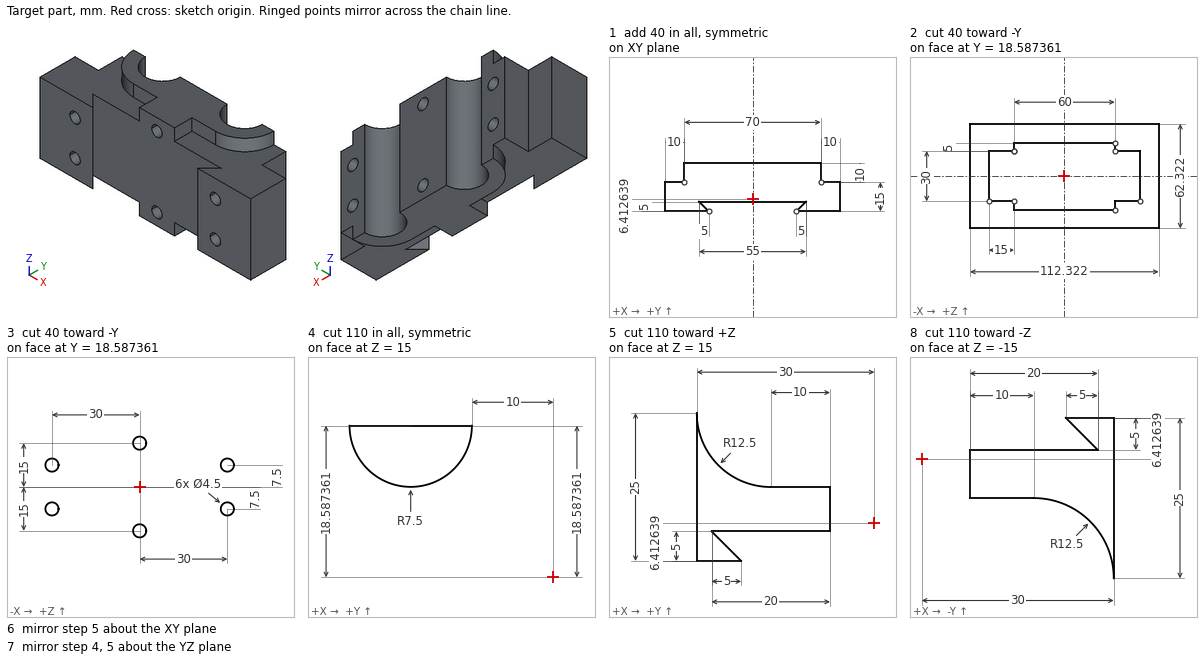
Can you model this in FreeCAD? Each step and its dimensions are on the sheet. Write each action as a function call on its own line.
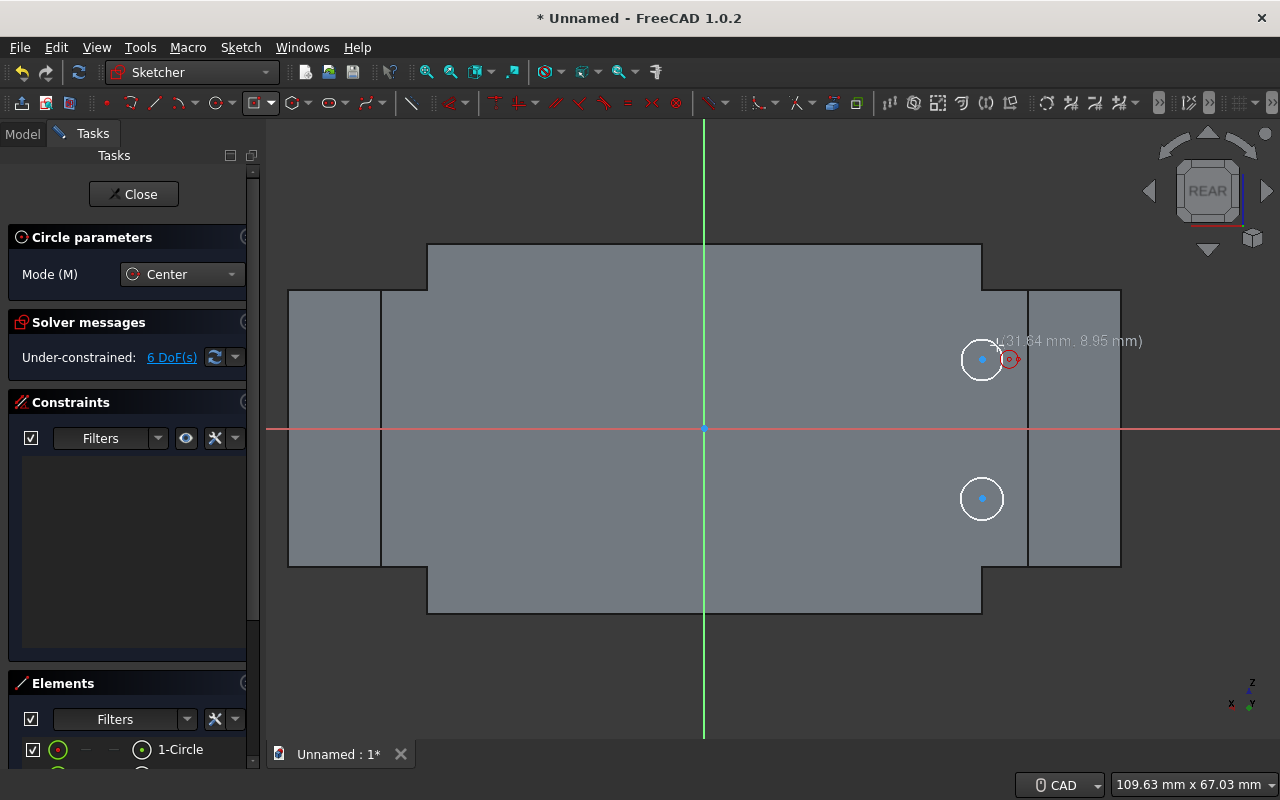
click(427, 359)
click(442, 345)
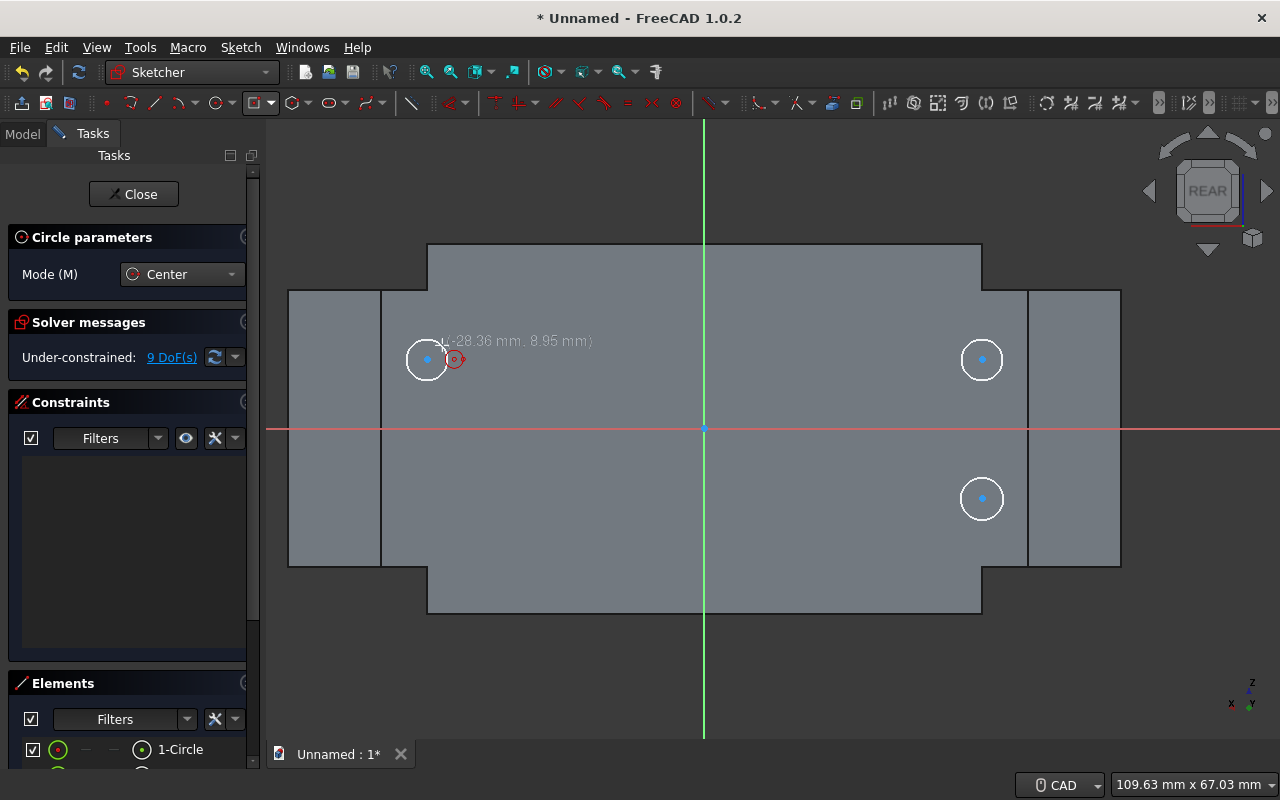
click(427, 498)
click(442, 483)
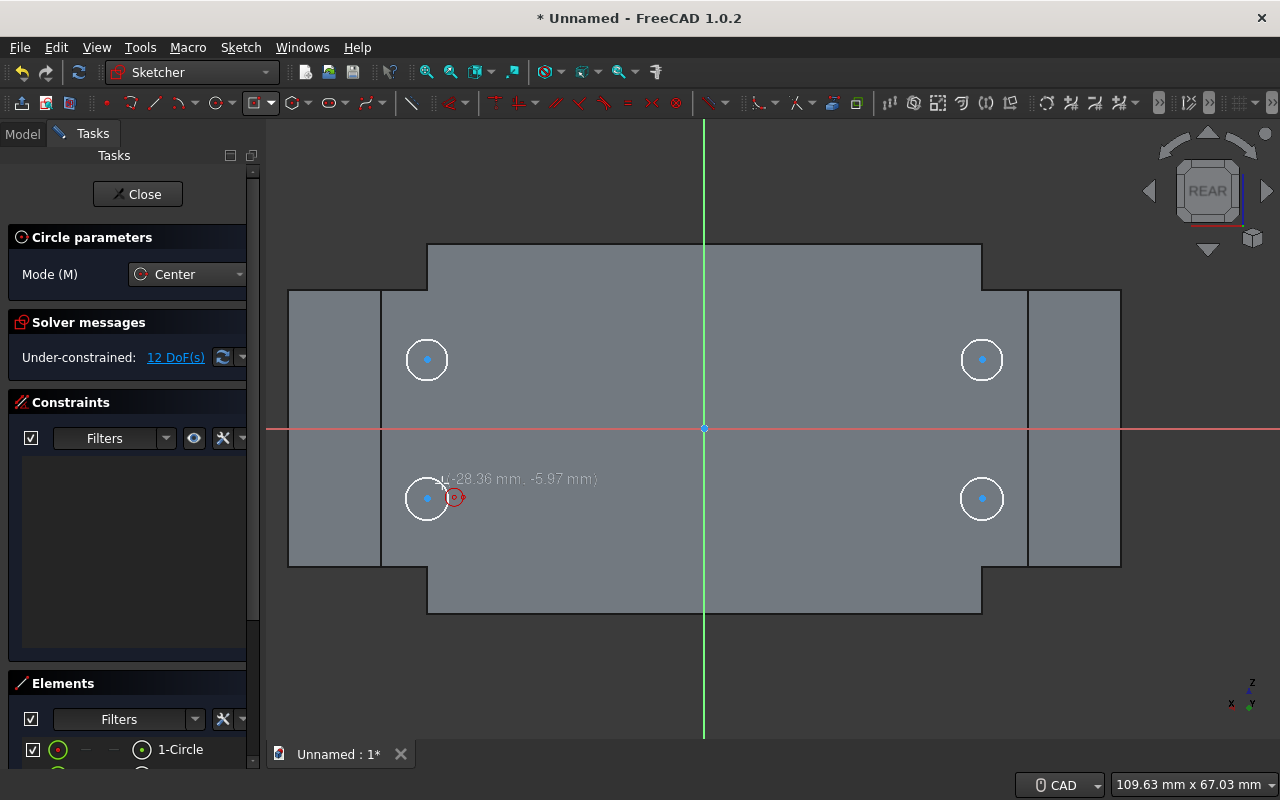
click(704, 567)
click(719, 553)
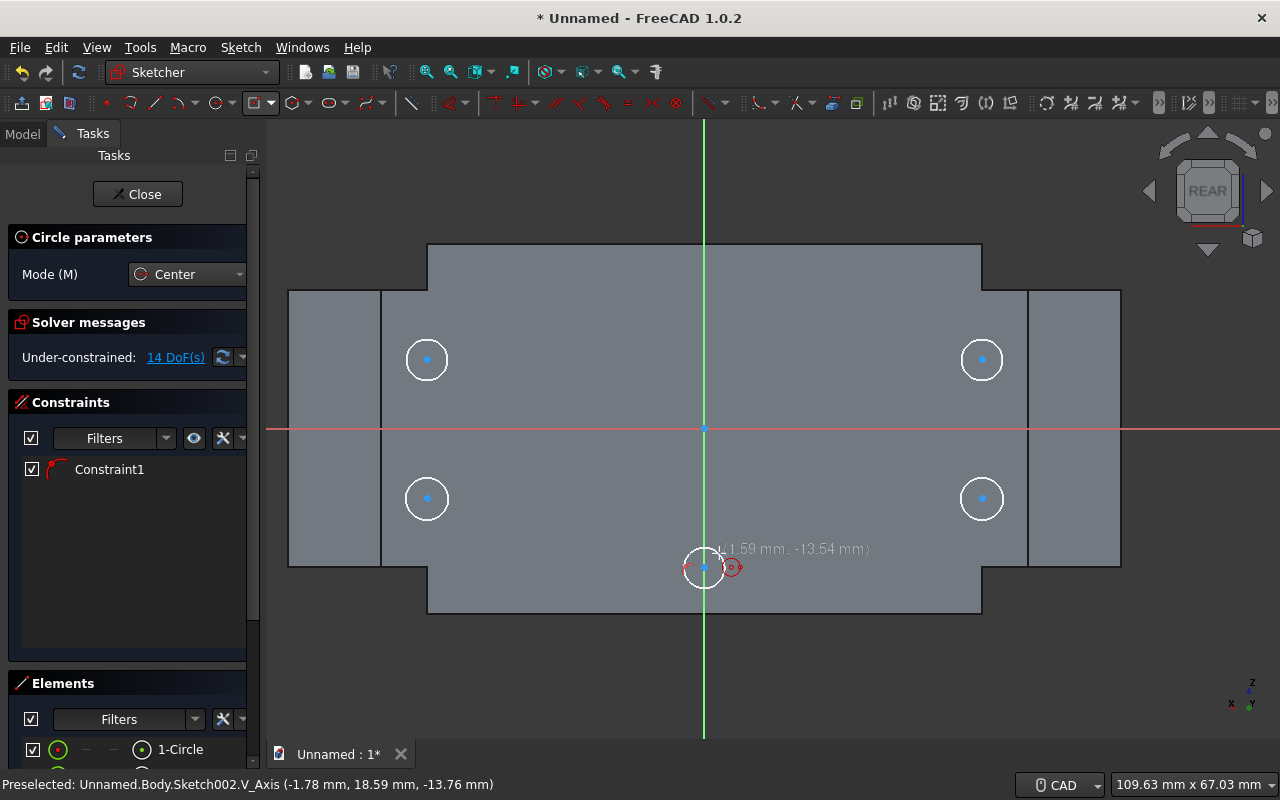
click(704, 290)
click(719, 275)
key(Escape)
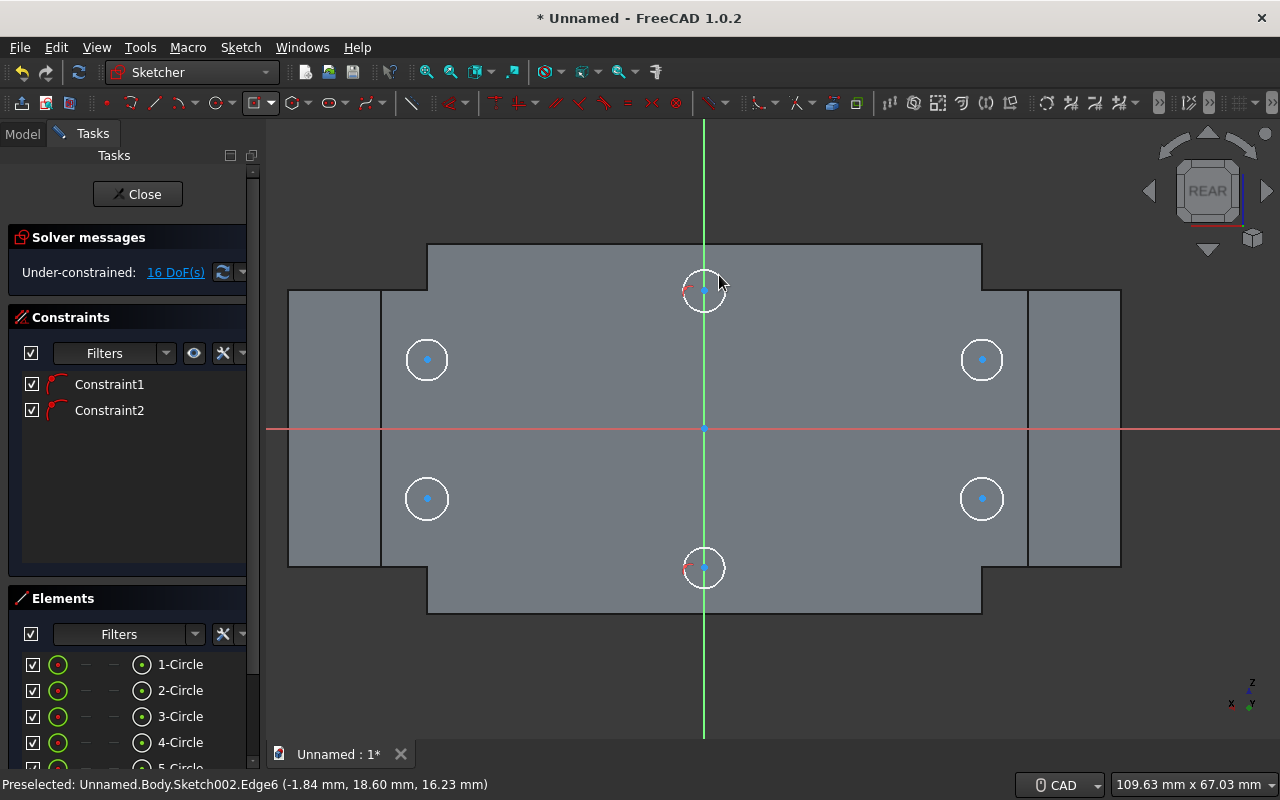
click(997, 484)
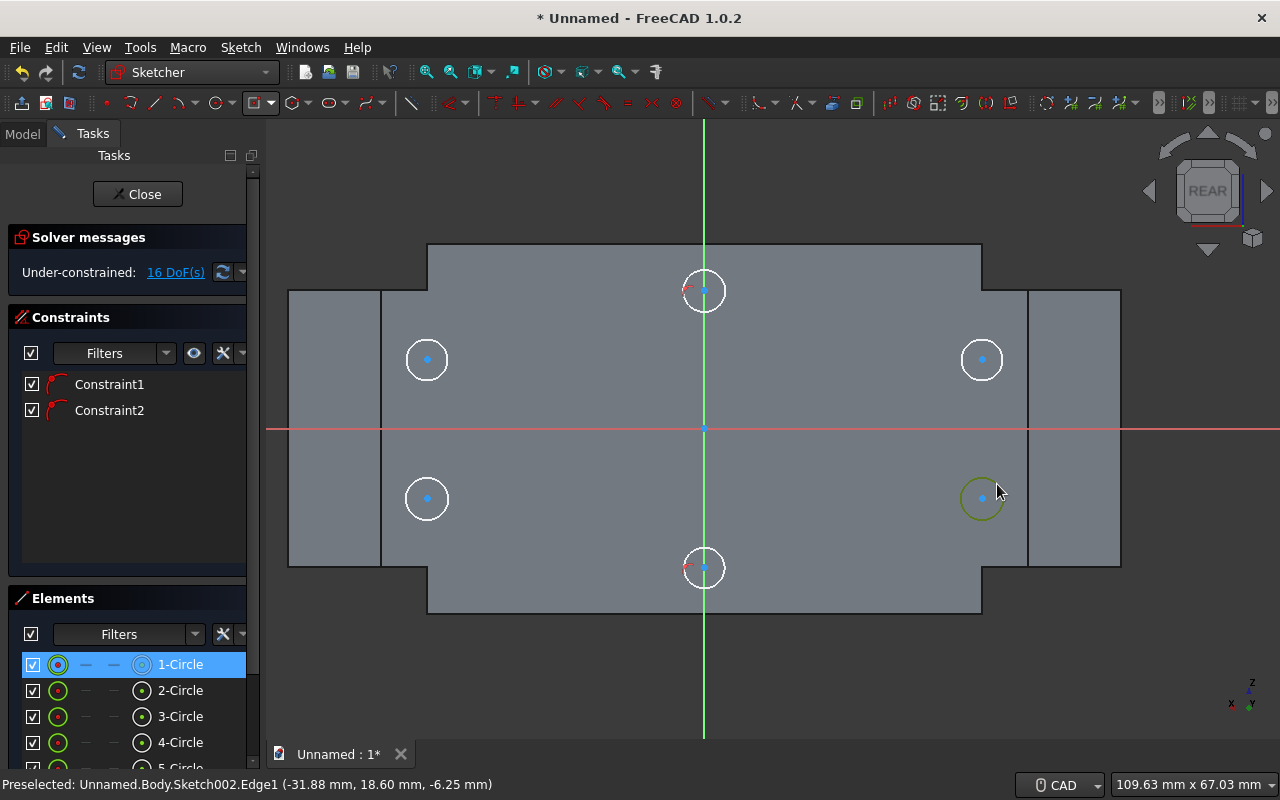
click(996, 345)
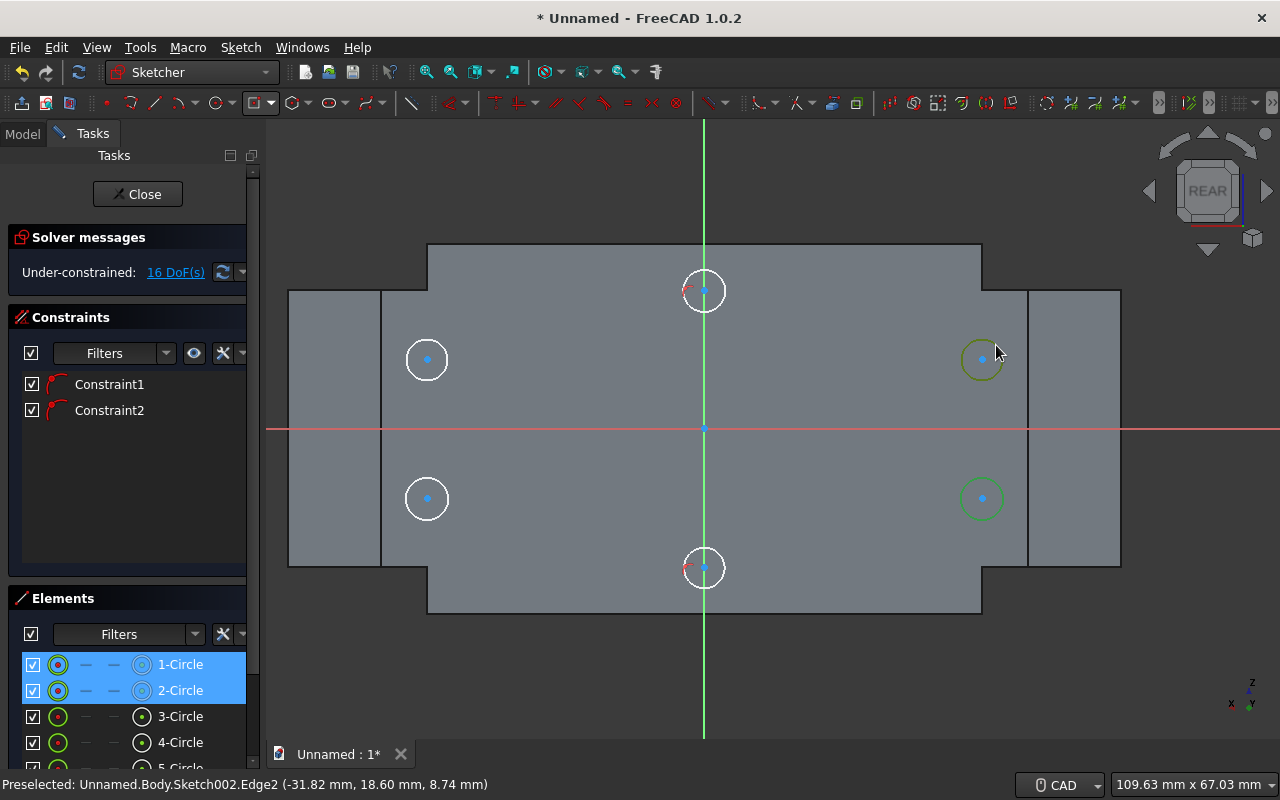
click(441, 345)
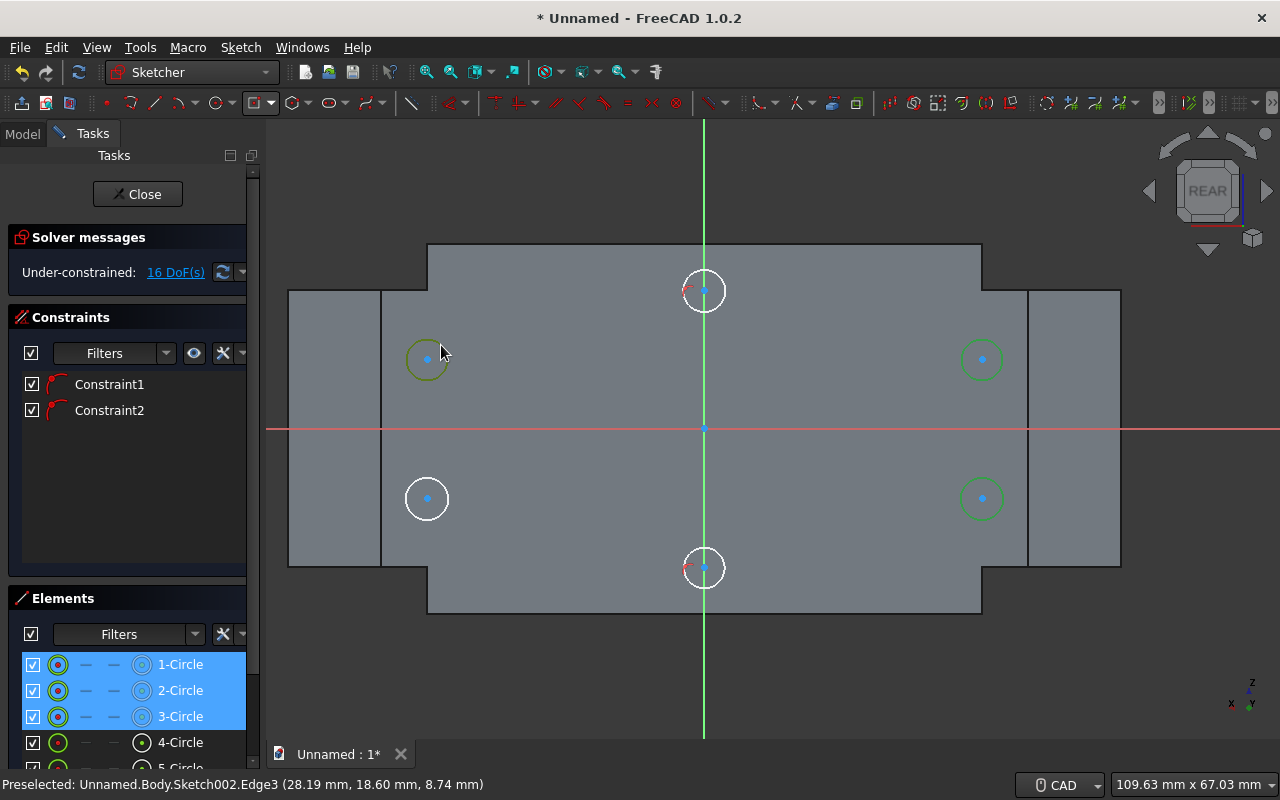
click(442, 484)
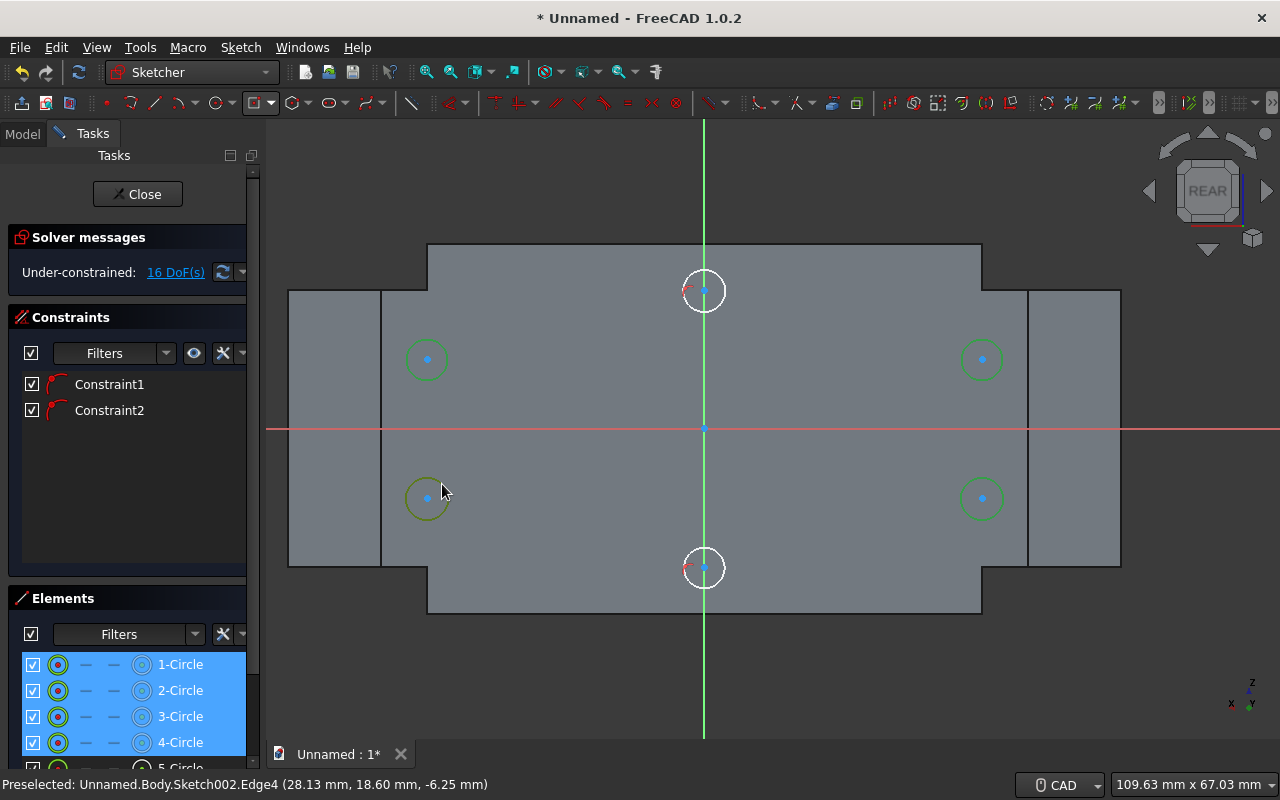
click(719, 554)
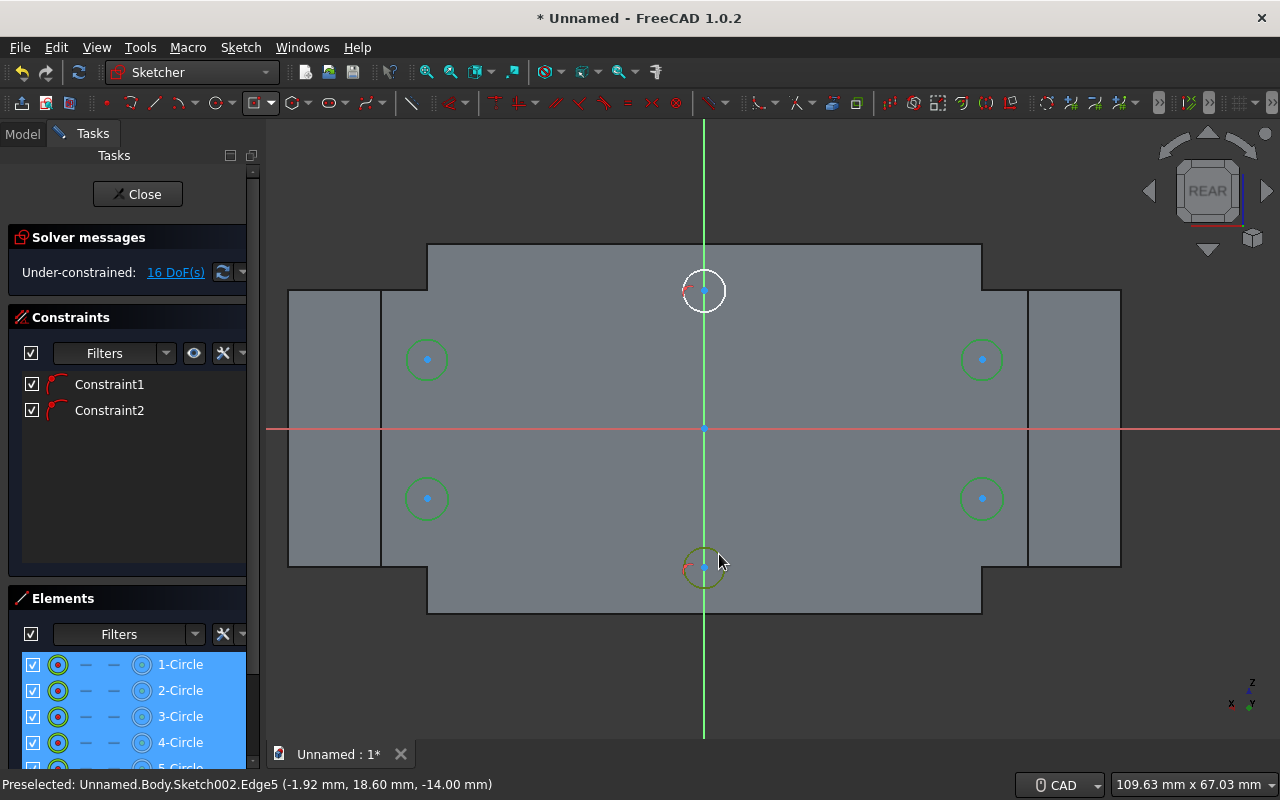
click(719, 276)